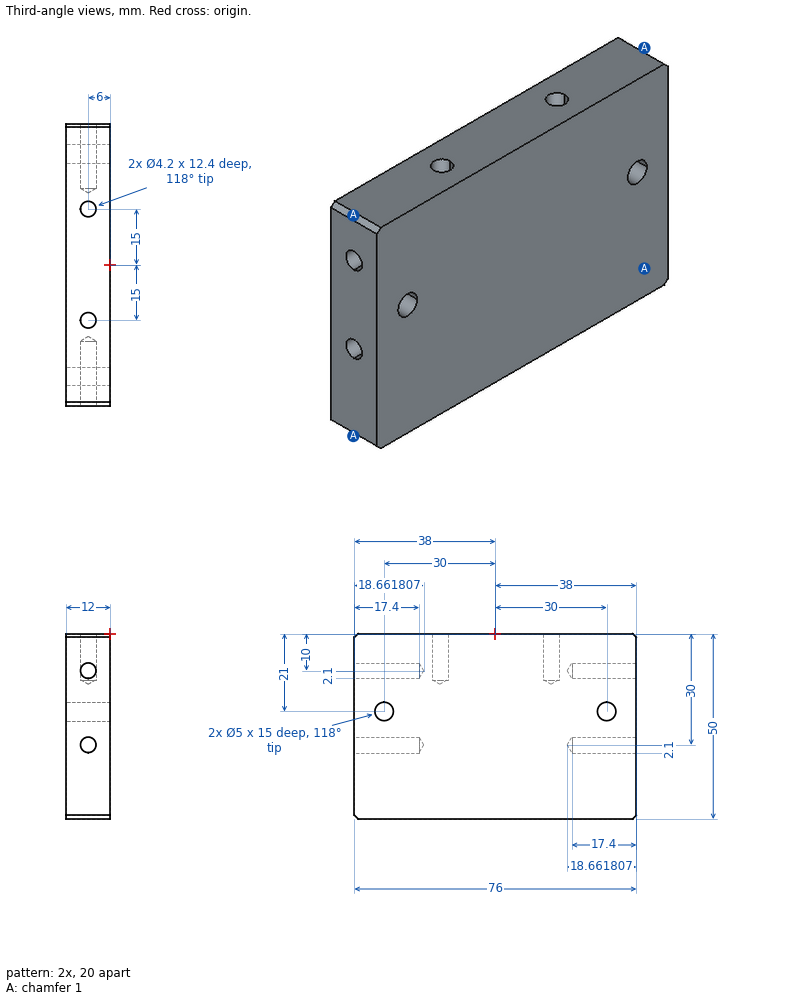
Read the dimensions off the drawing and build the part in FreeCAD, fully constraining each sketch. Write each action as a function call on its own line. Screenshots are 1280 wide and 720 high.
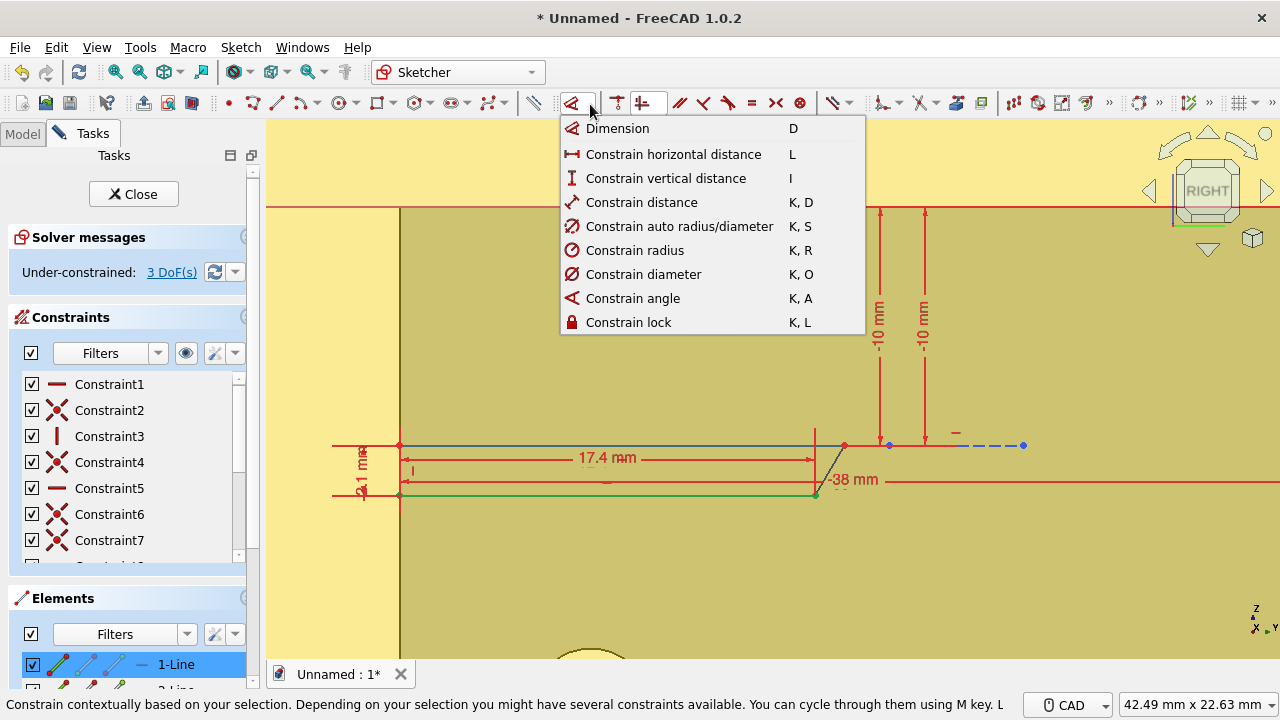
click(713, 154)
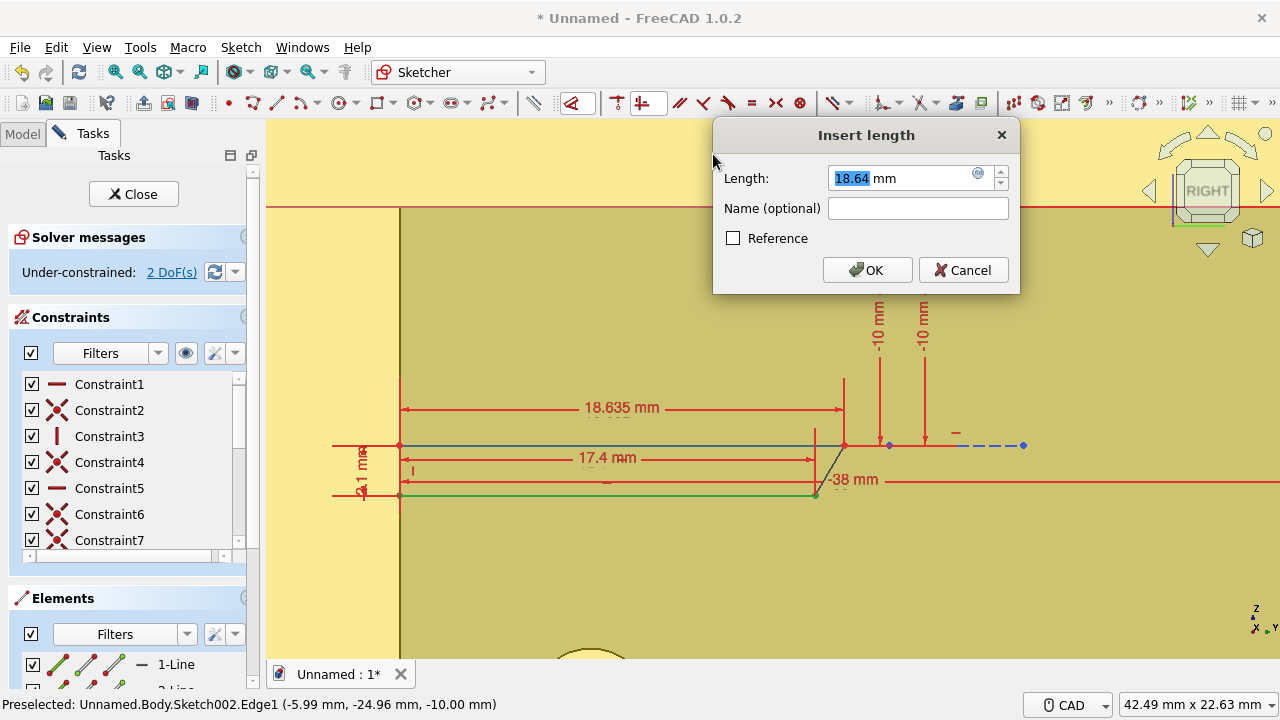
text(18.661807)
key(Return)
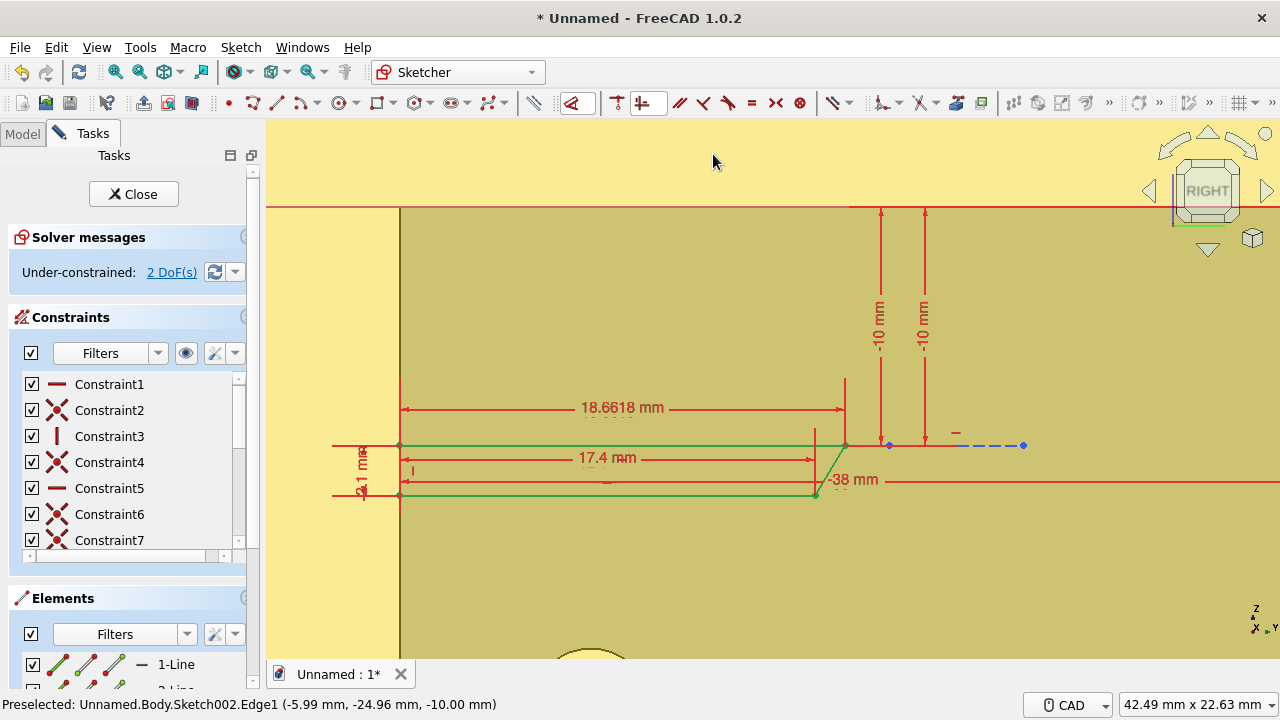
click(134, 194)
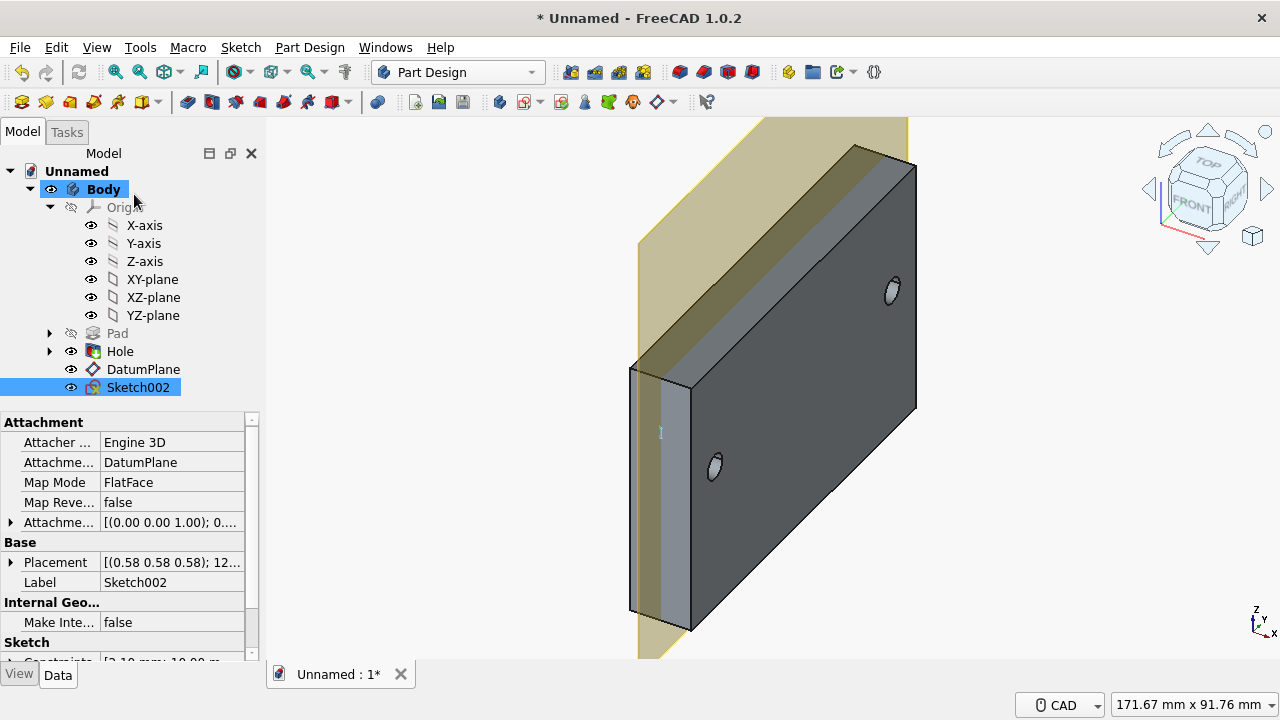
click(236, 102)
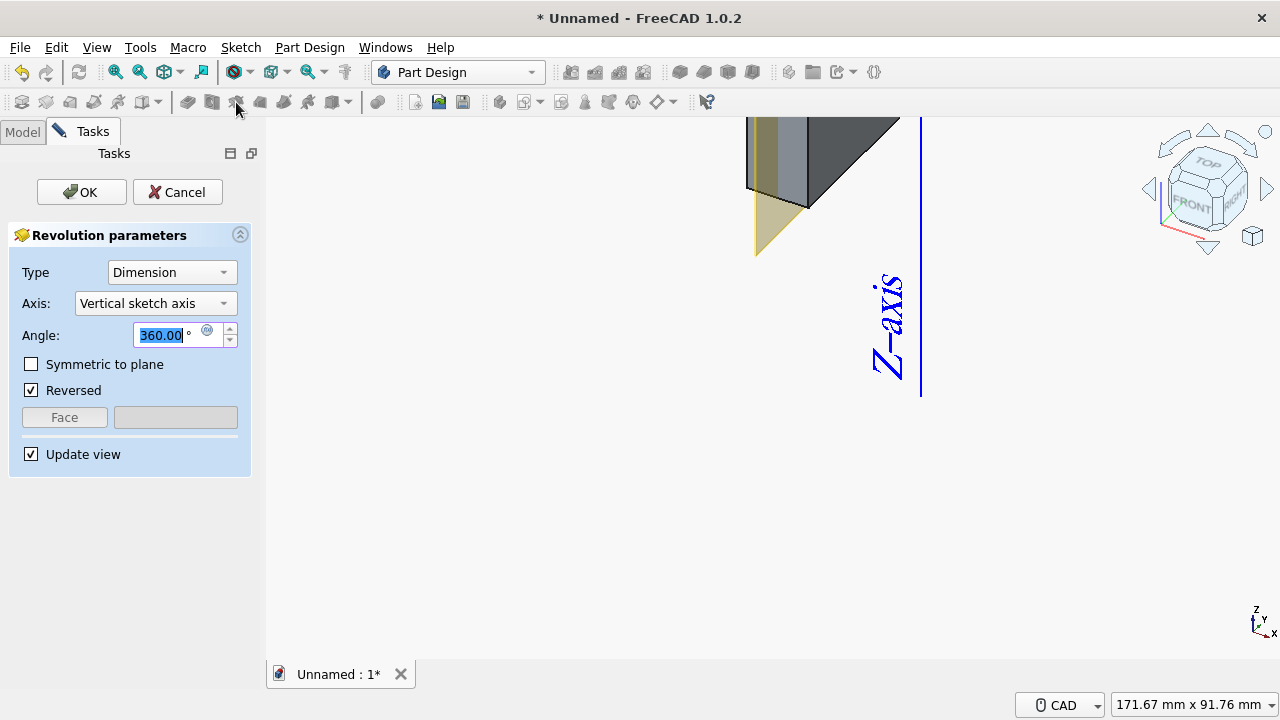
click(156, 304)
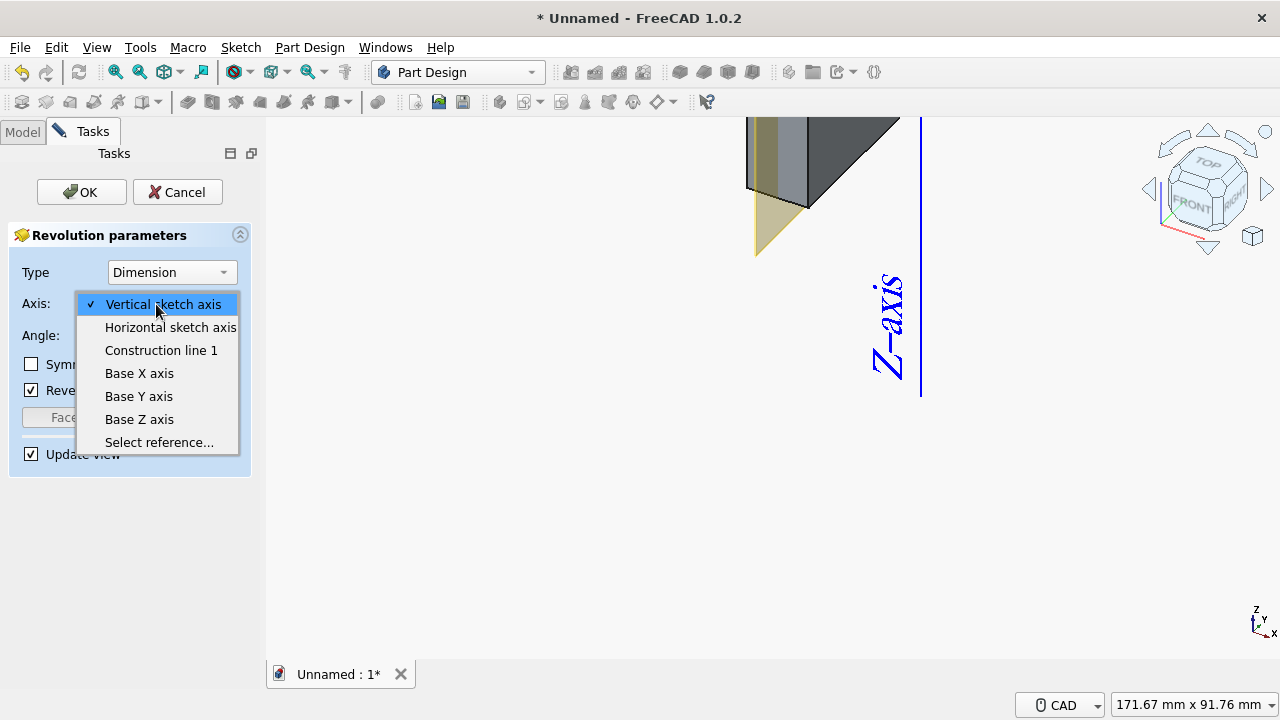
click(156, 350)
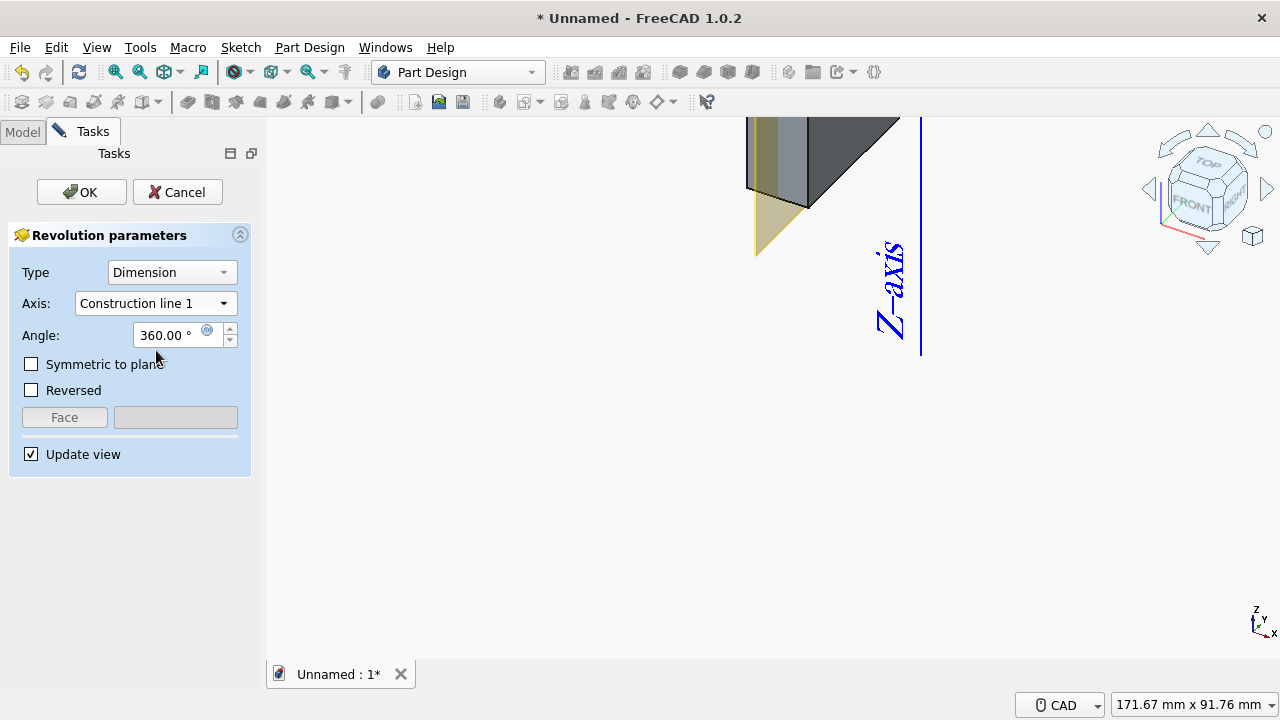
click(82, 192)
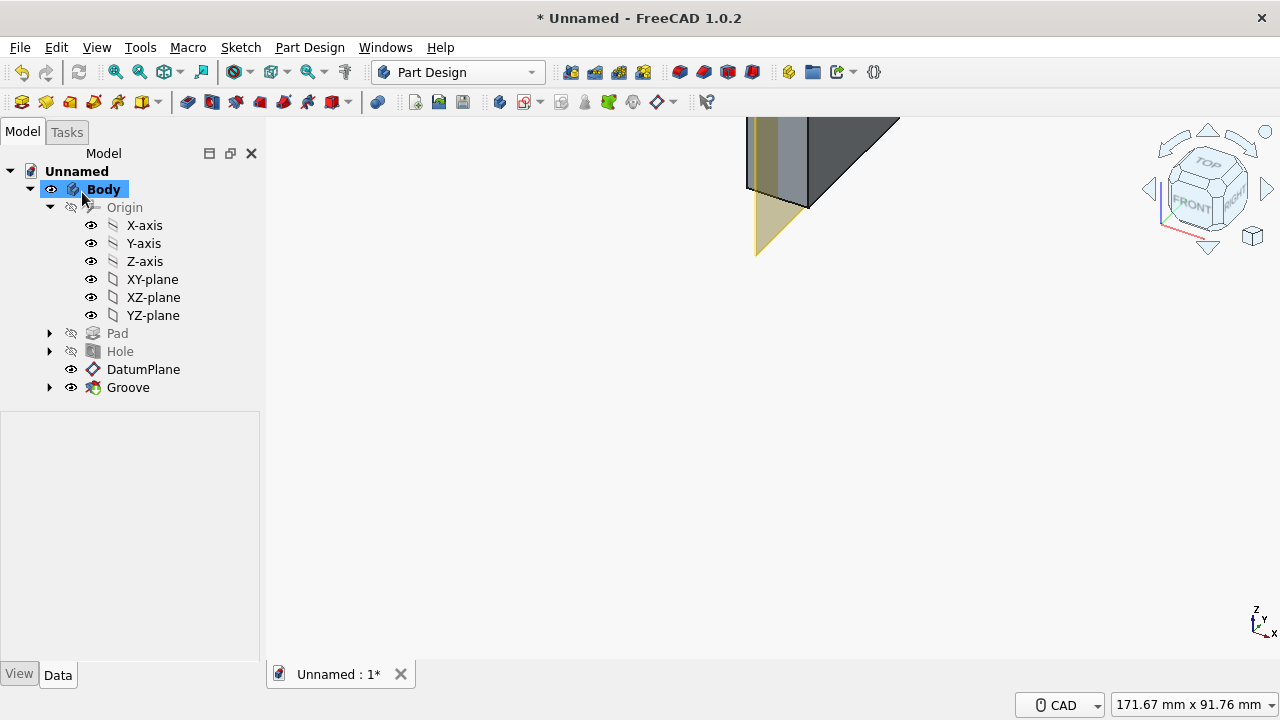
click(116, 369)
key(space)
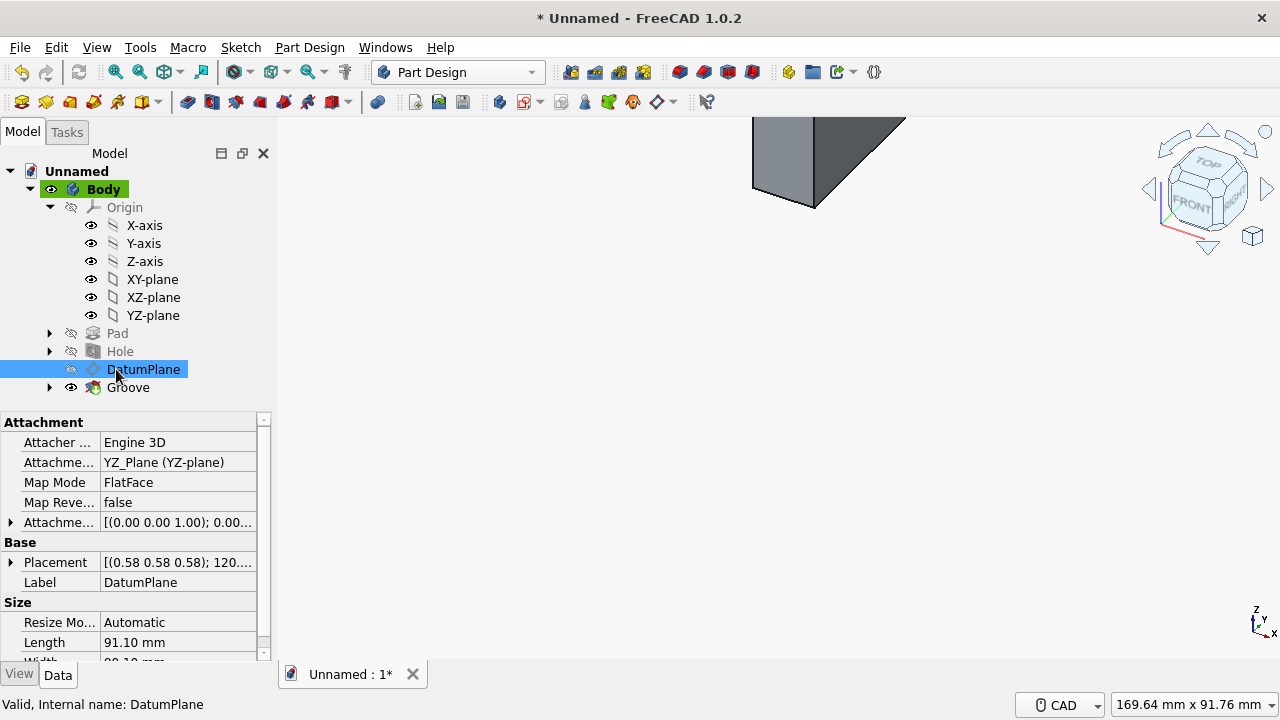
key(v)
key(f)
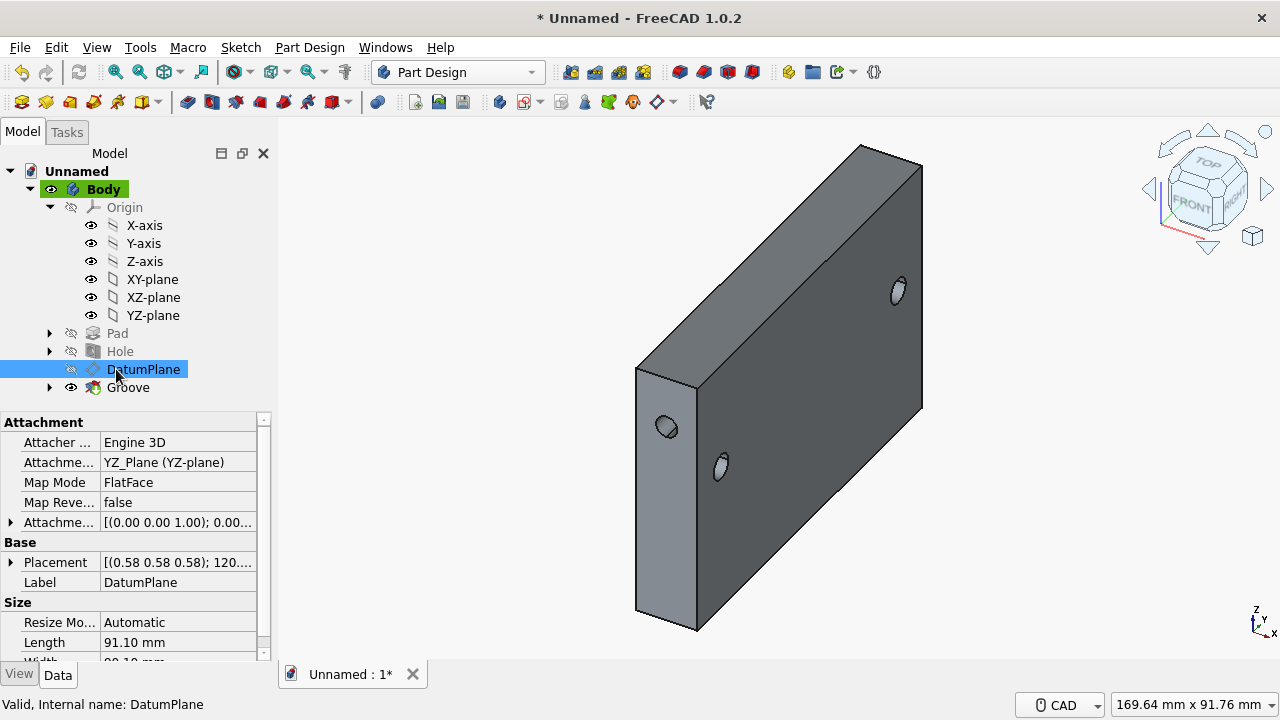
click(116, 387)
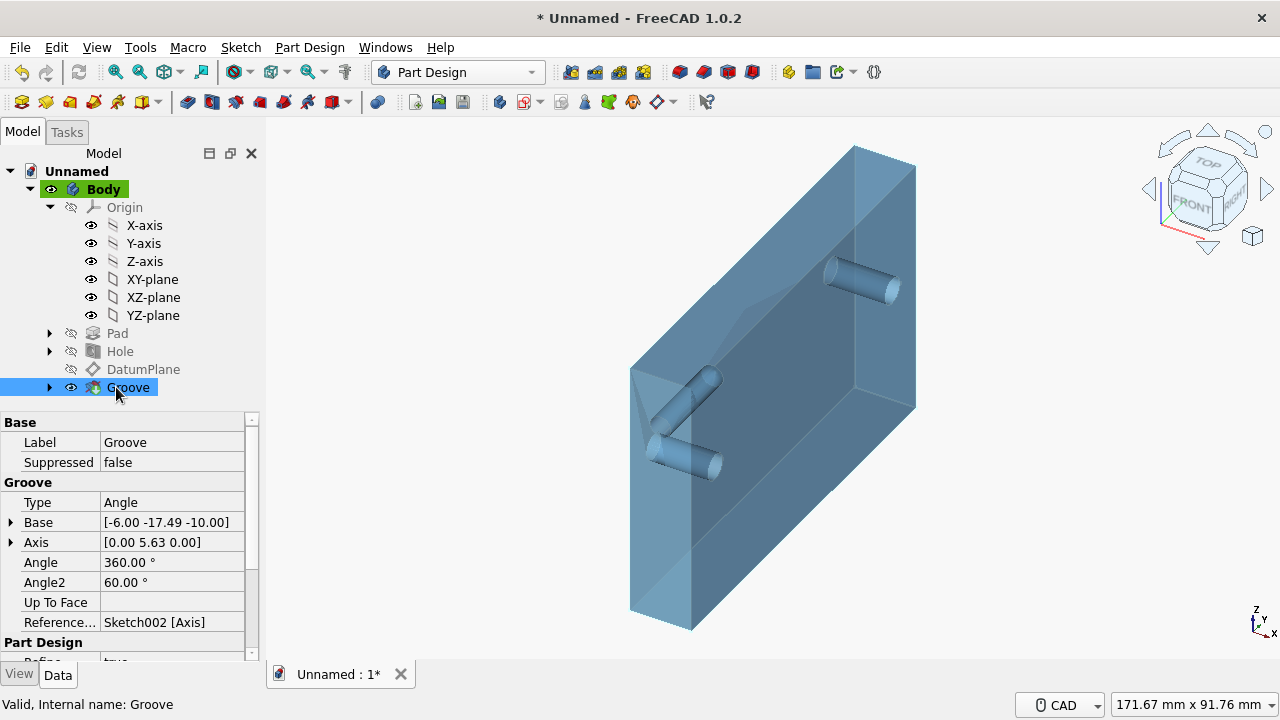
click(596, 72)